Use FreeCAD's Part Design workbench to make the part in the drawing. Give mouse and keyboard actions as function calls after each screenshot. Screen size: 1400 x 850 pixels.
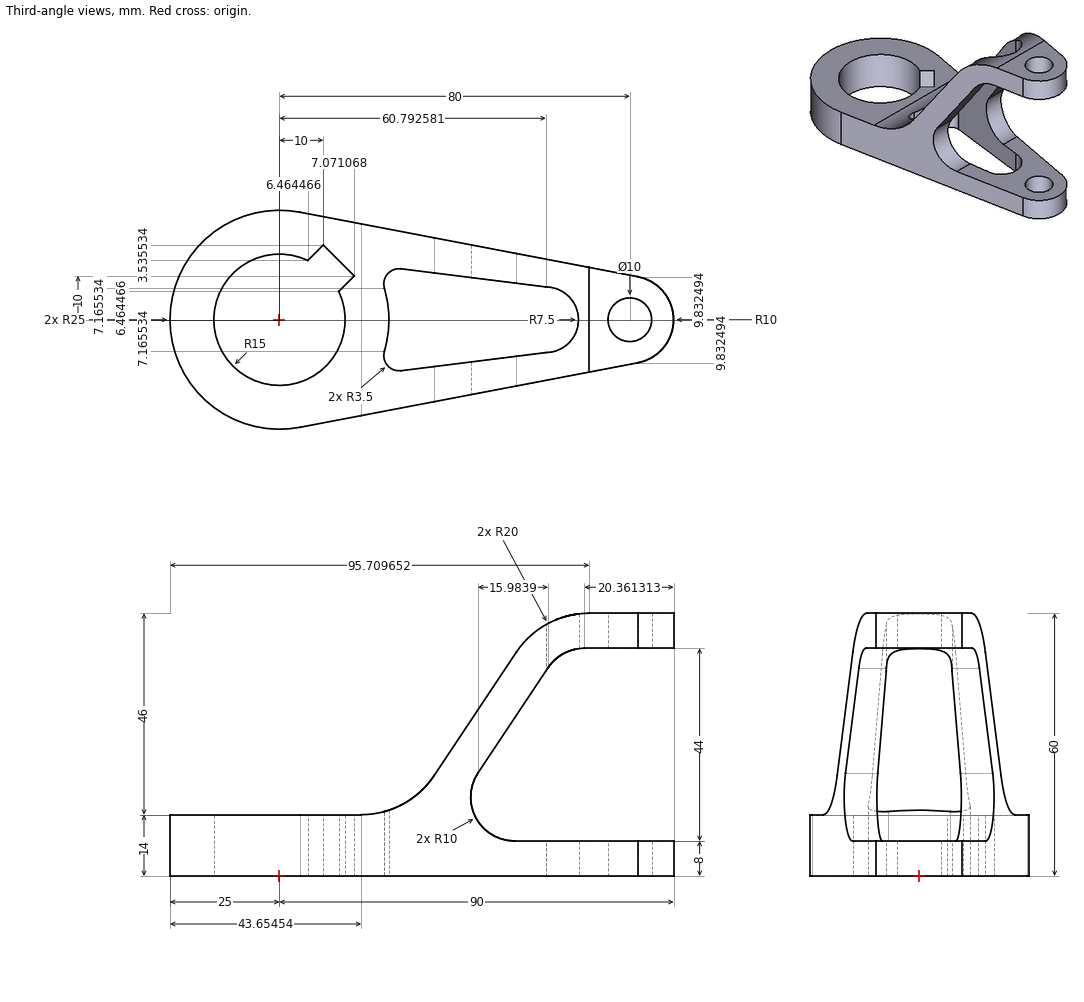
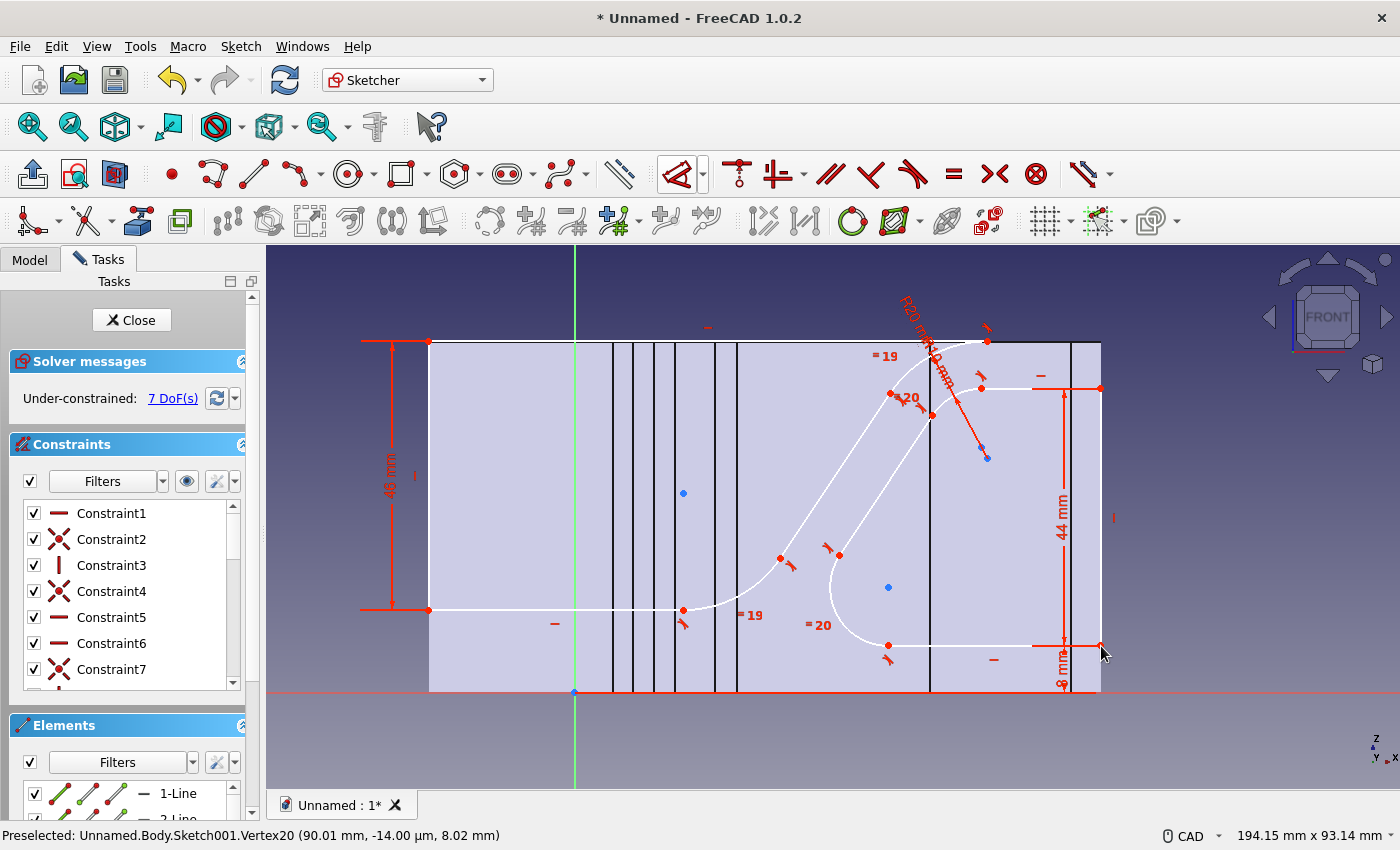
click(683, 610)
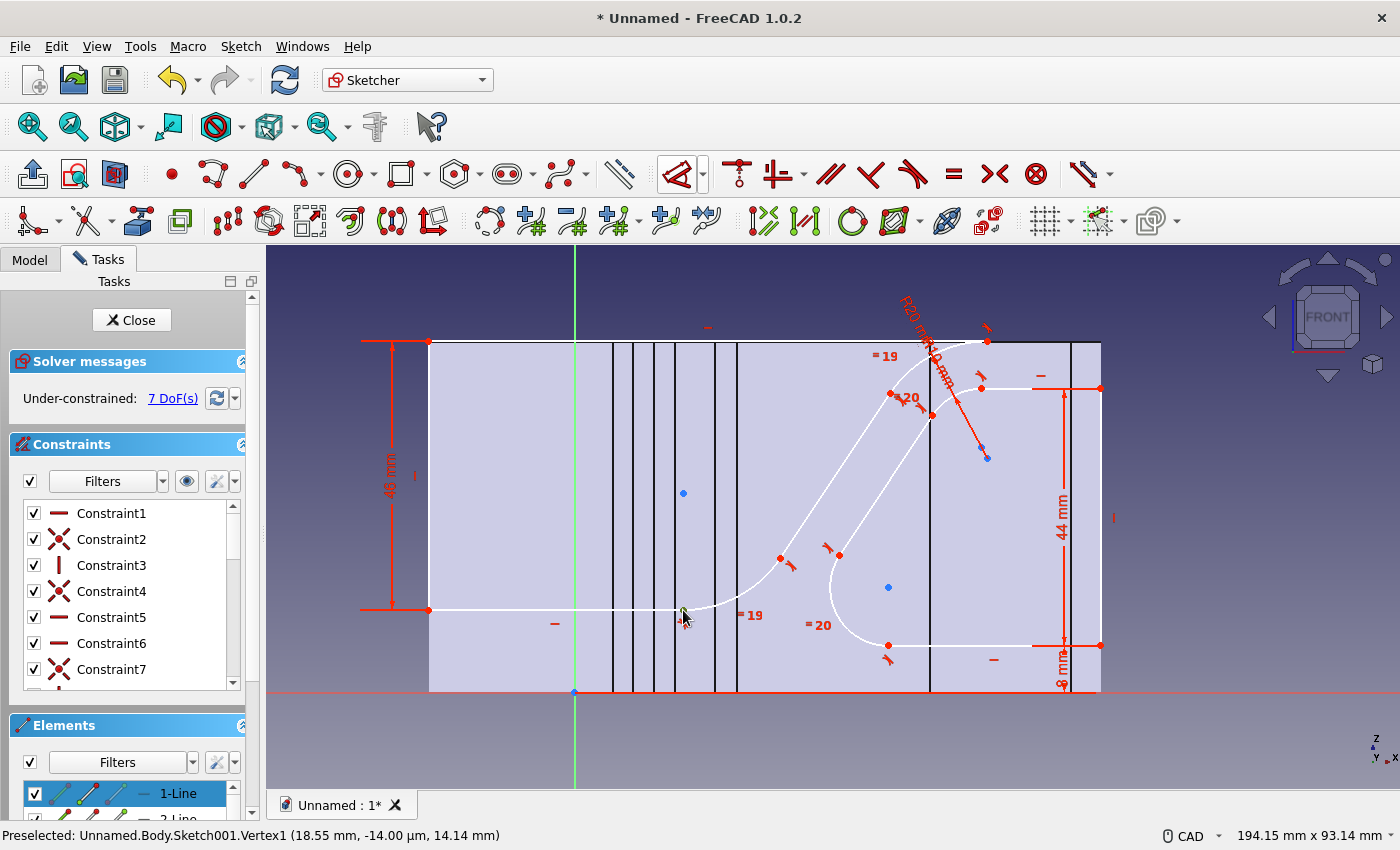
click(702, 174)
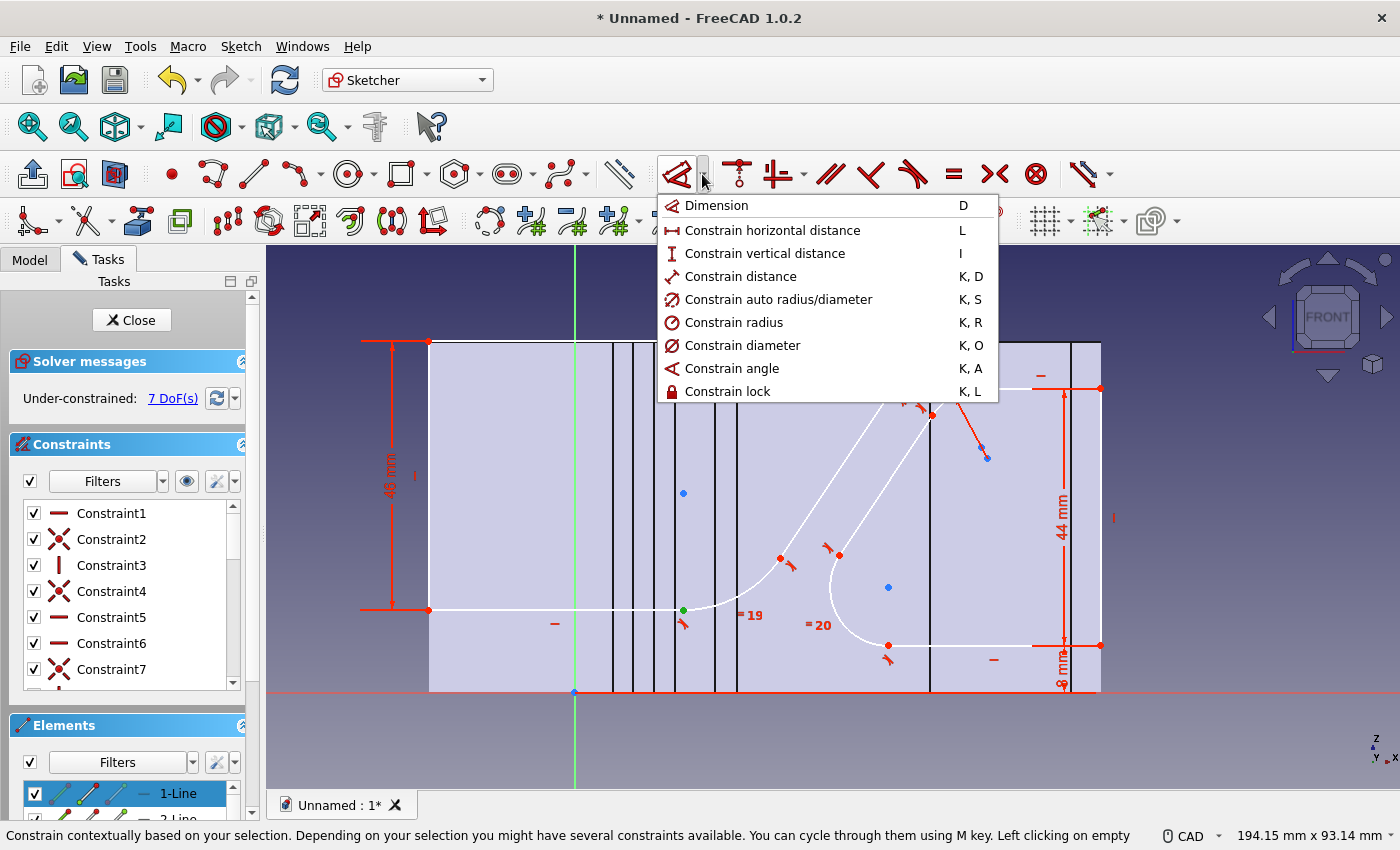
click(828, 254)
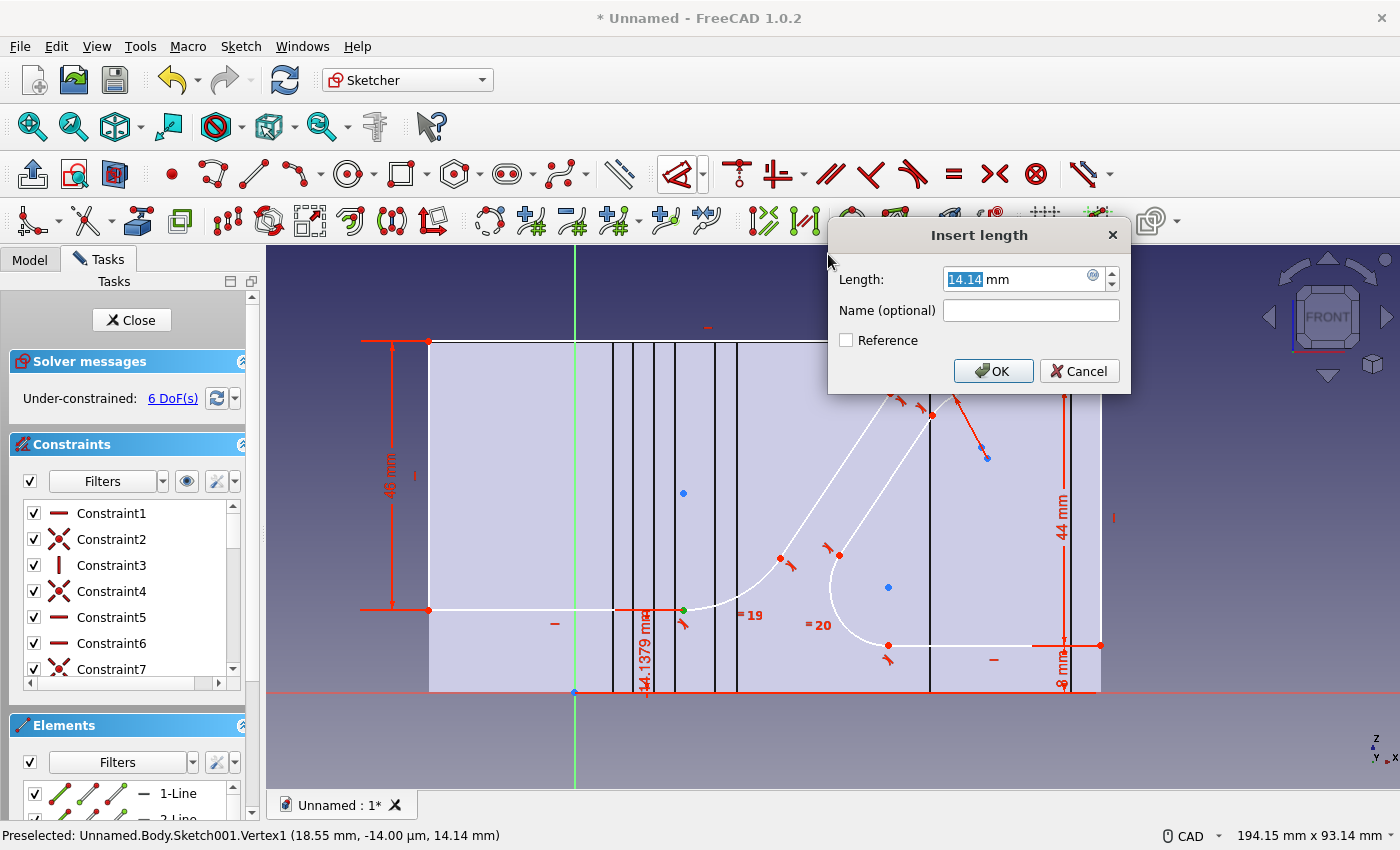
text(14)
key(Return)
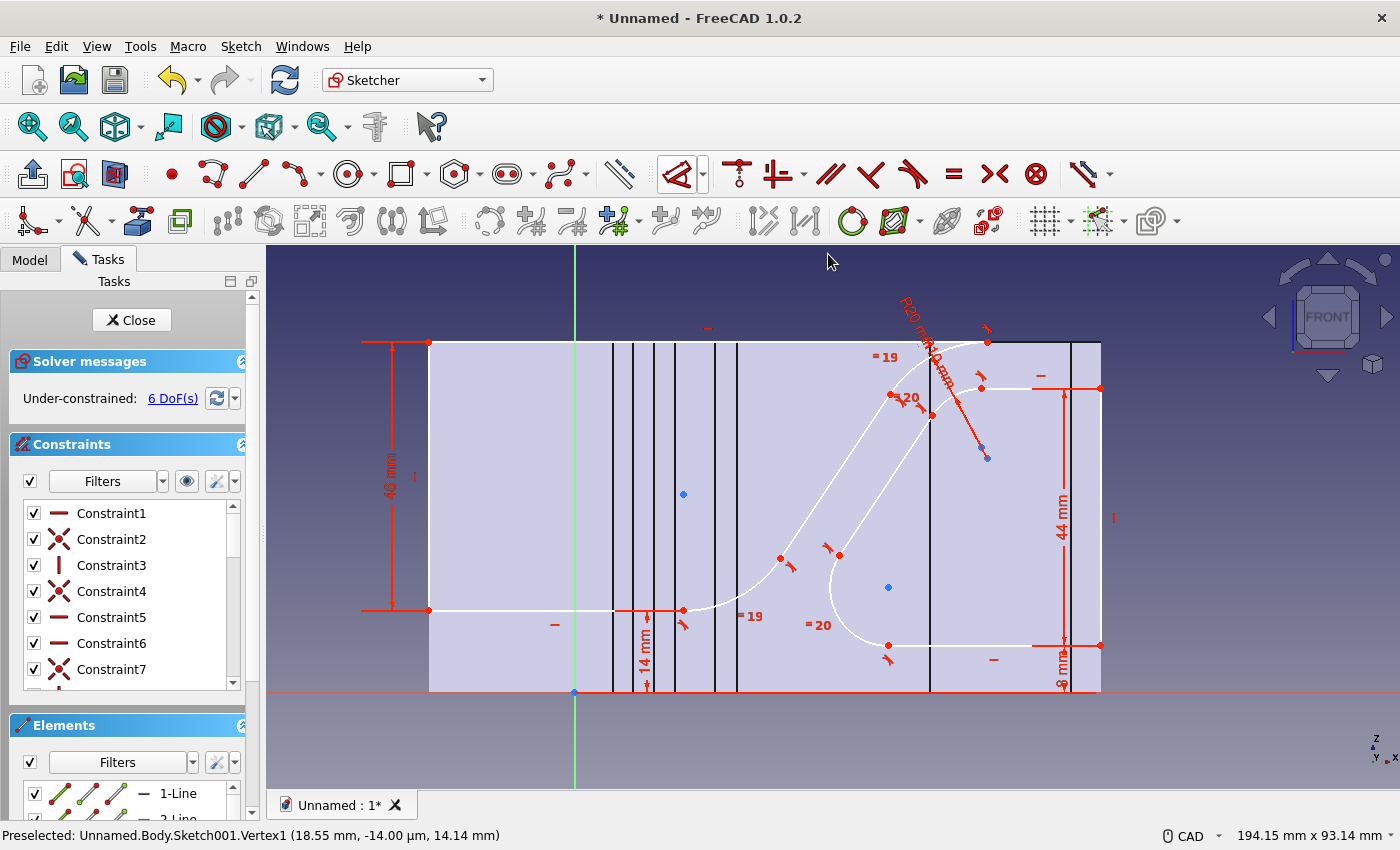
click(429, 611)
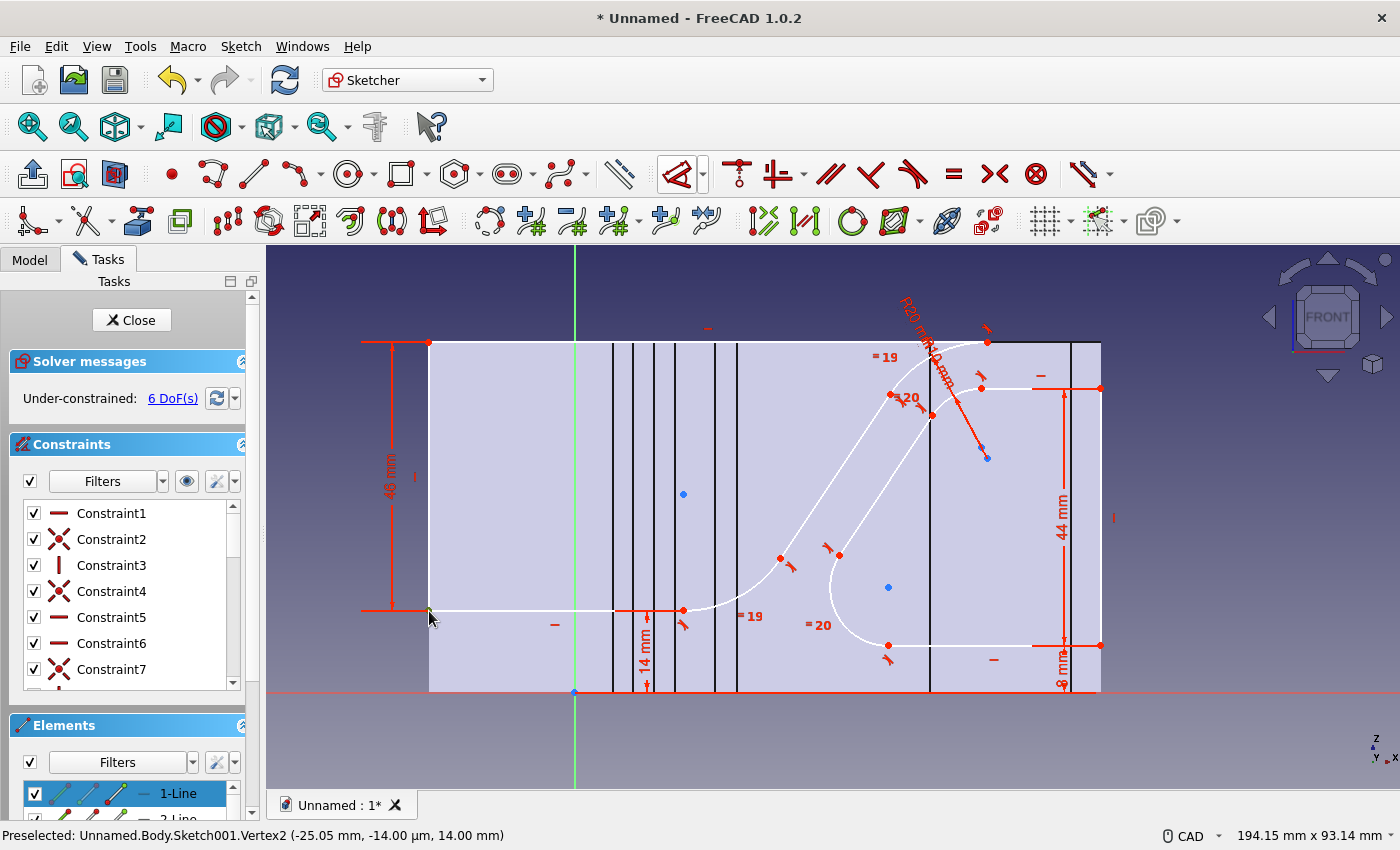
click(702, 174)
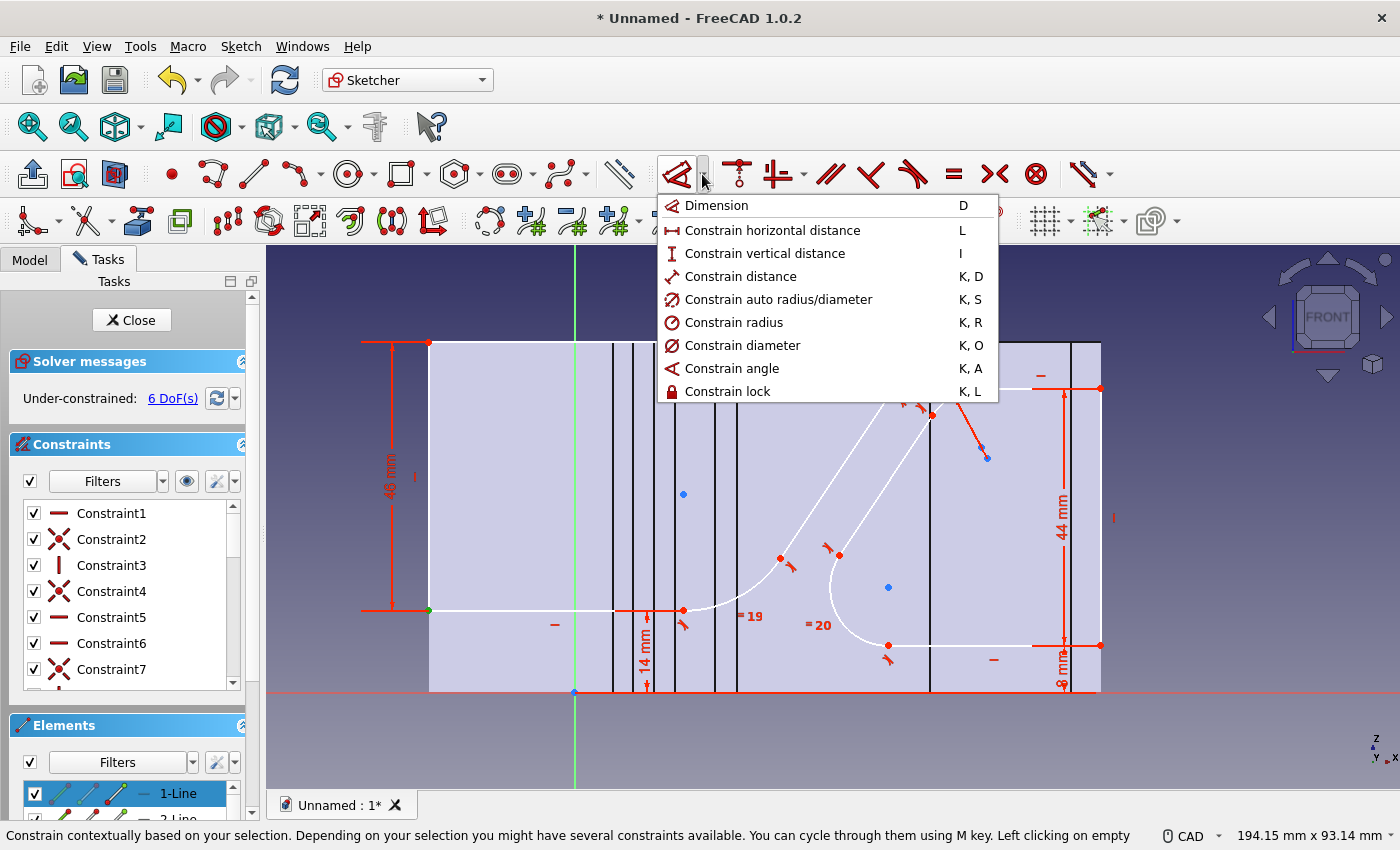
click(828, 230)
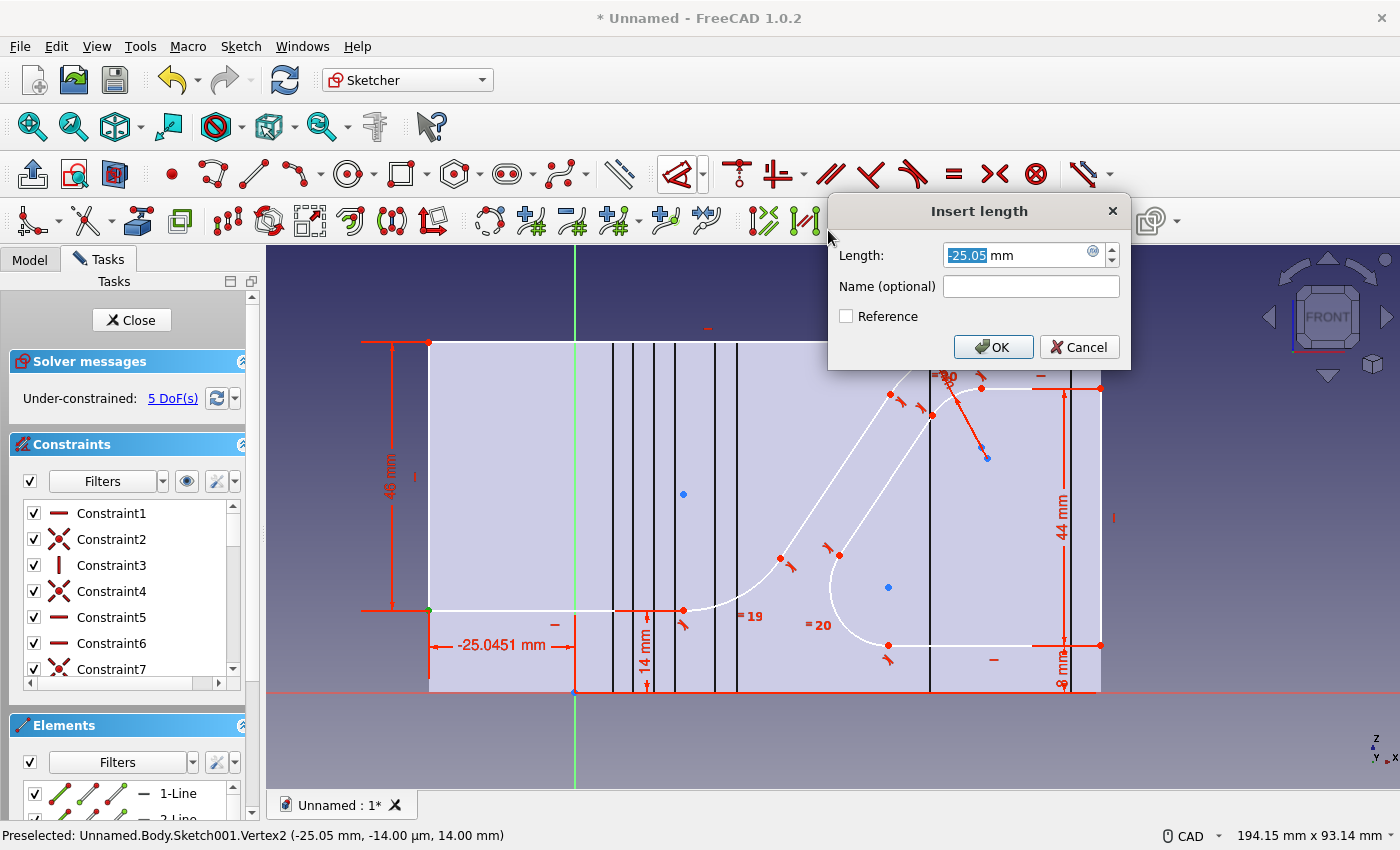
text(-25)
key(Return)